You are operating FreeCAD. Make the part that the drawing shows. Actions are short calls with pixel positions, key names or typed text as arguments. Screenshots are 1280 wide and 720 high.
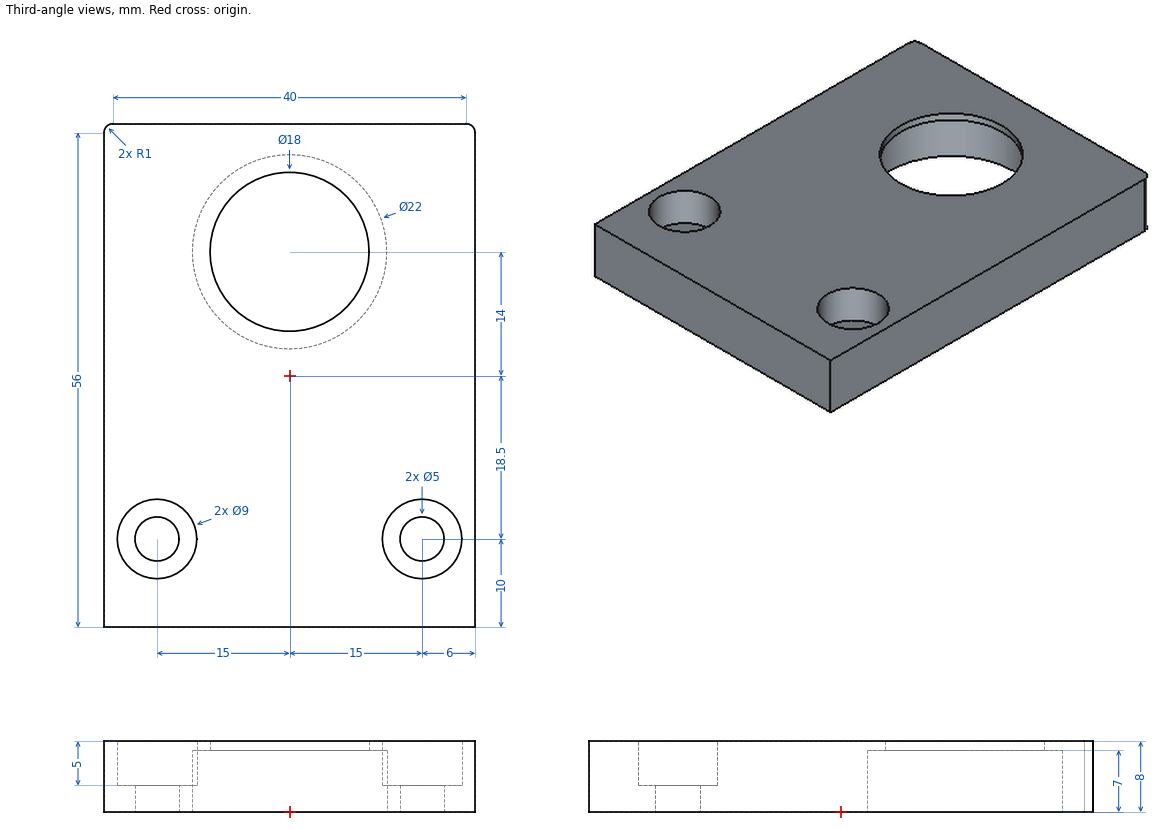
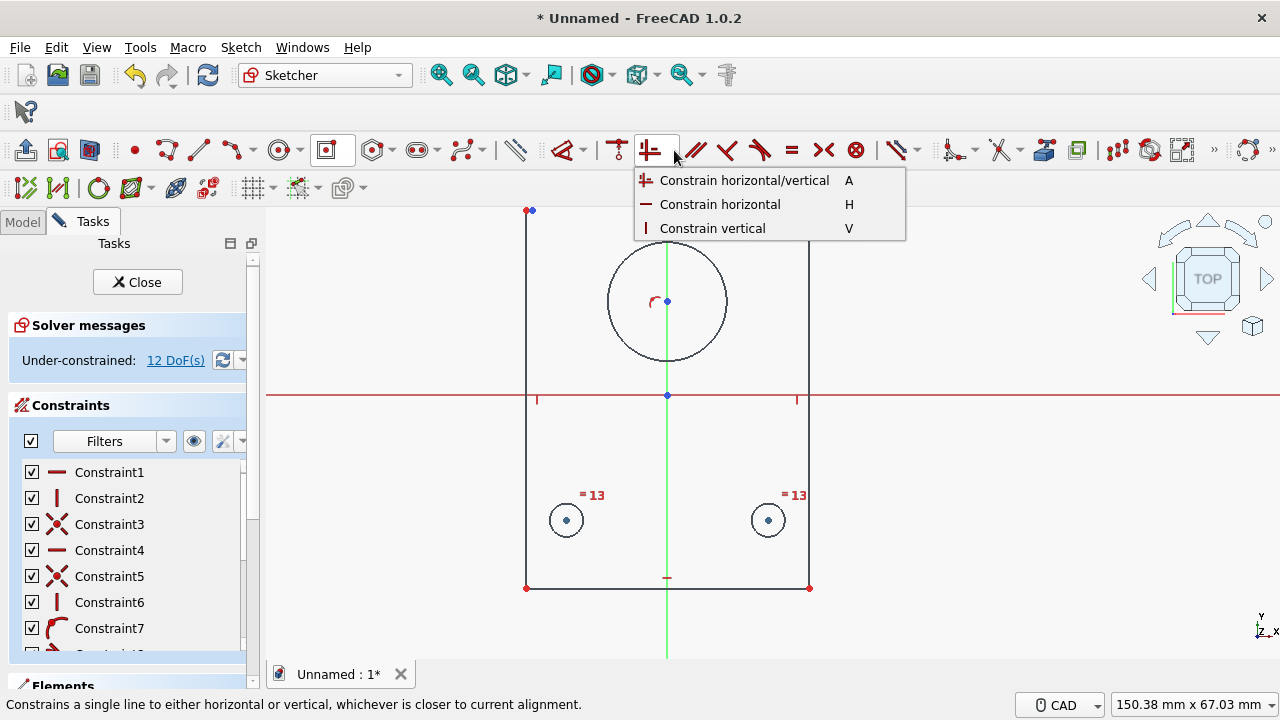
click(770, 204)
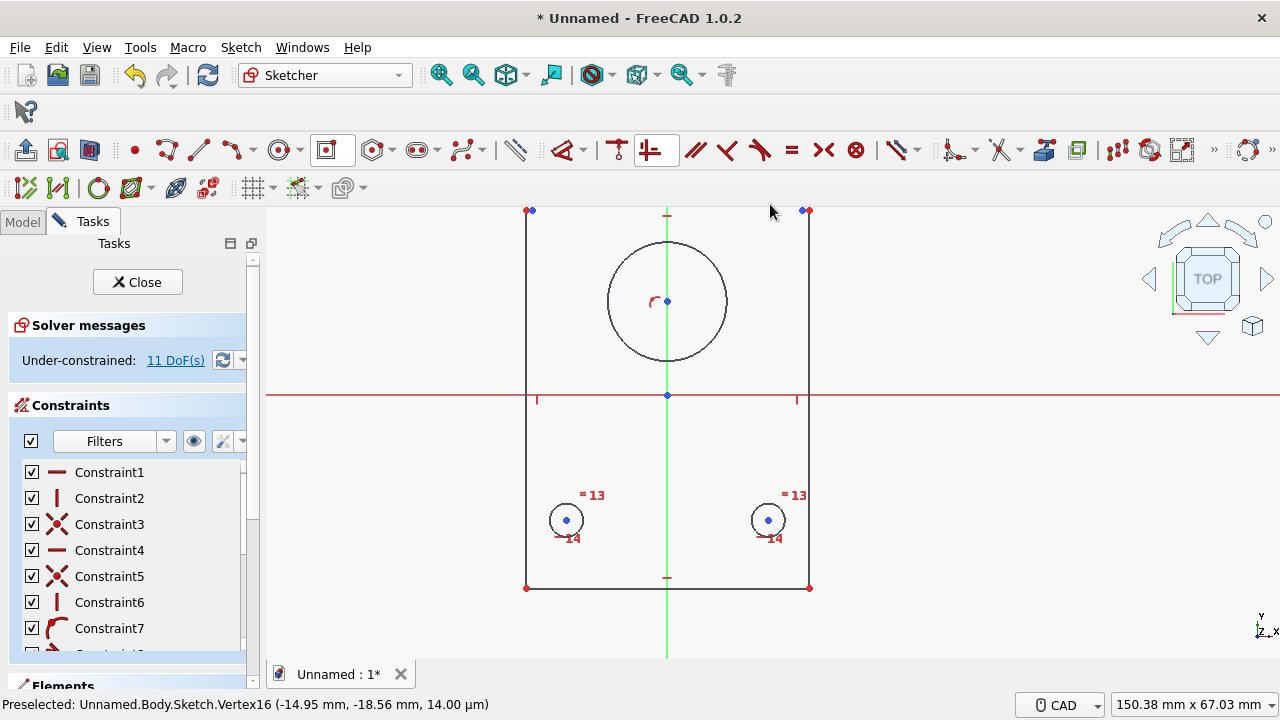
click(562, 150)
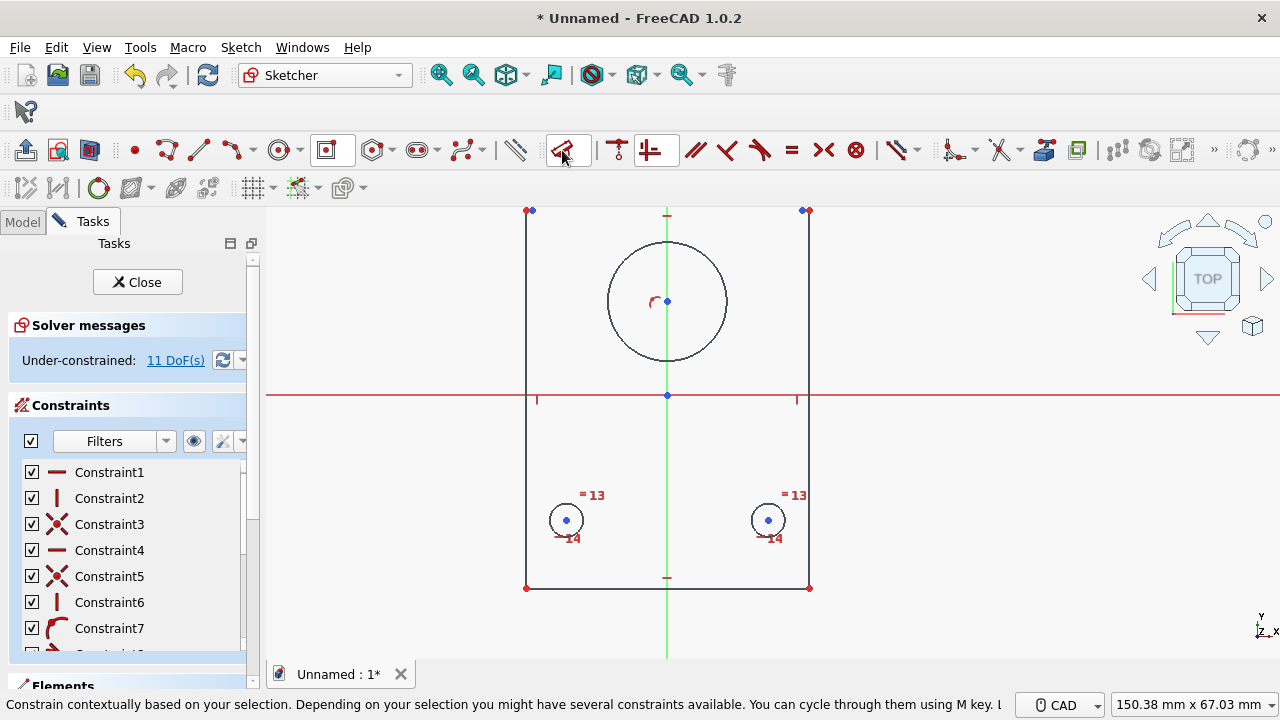
scroll(780, 510, down, 2)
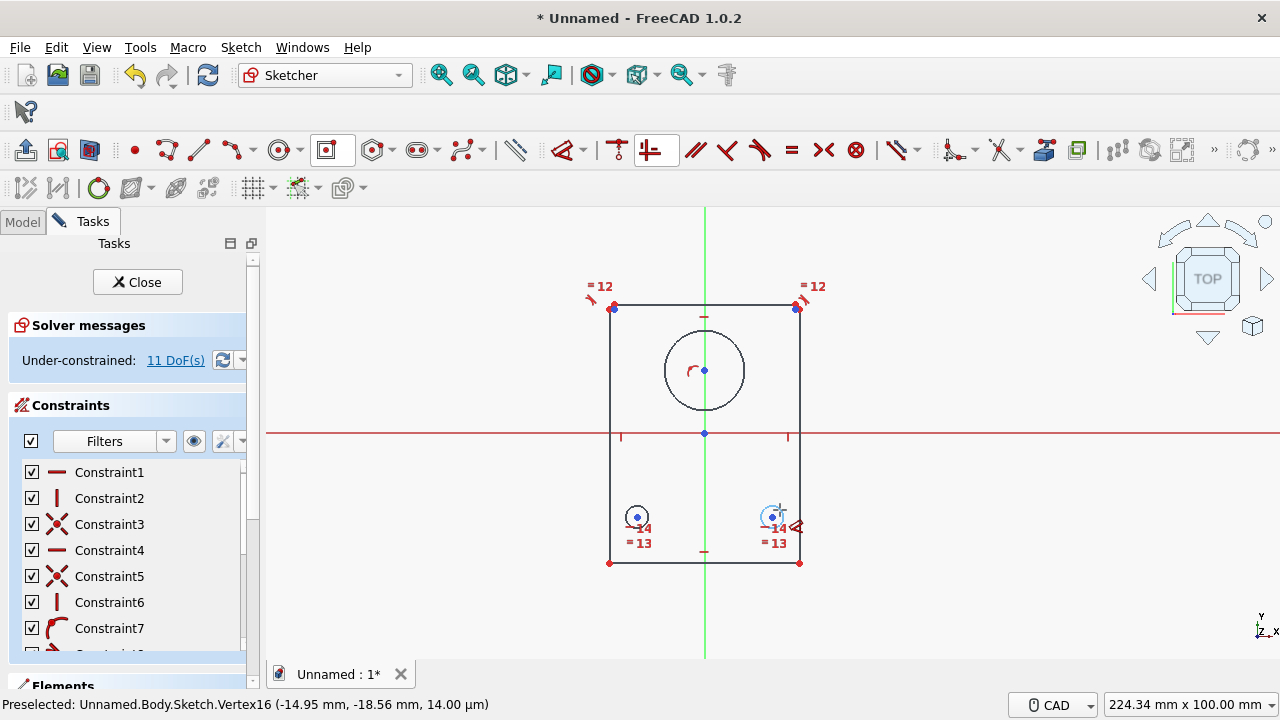
scroll(611, 306, up, 11)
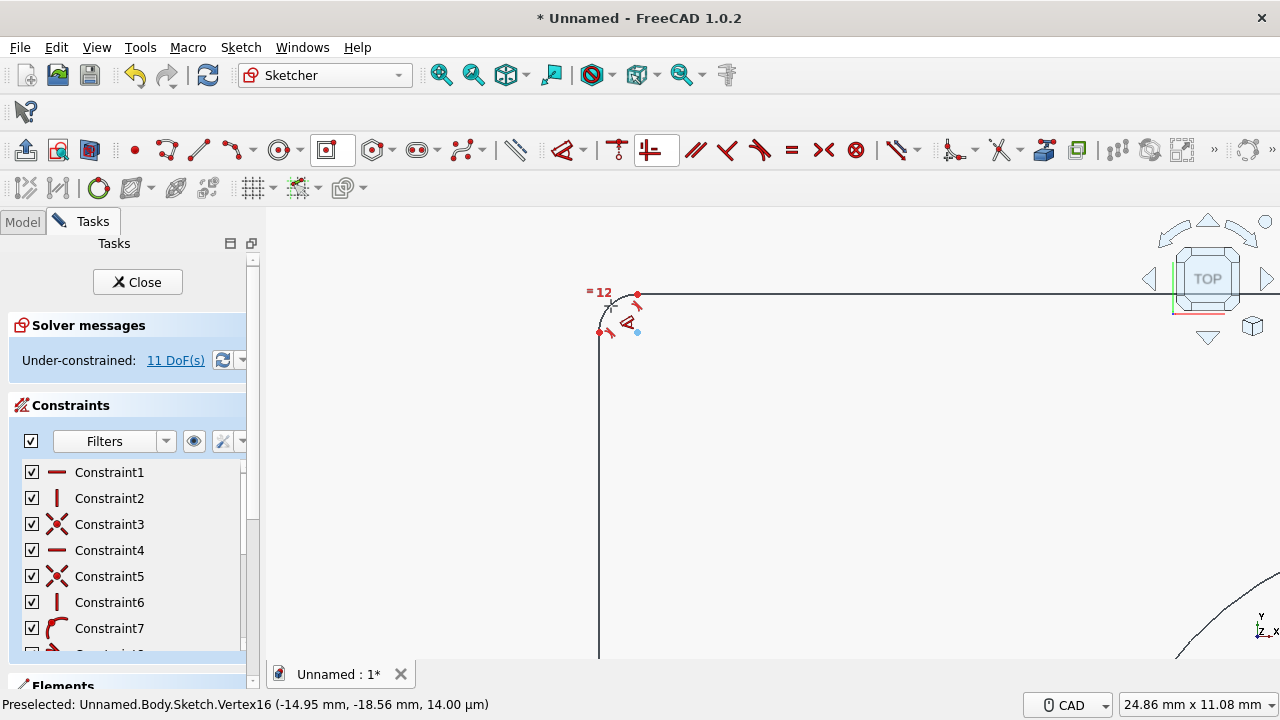
click(610, 306)
click(587, 284)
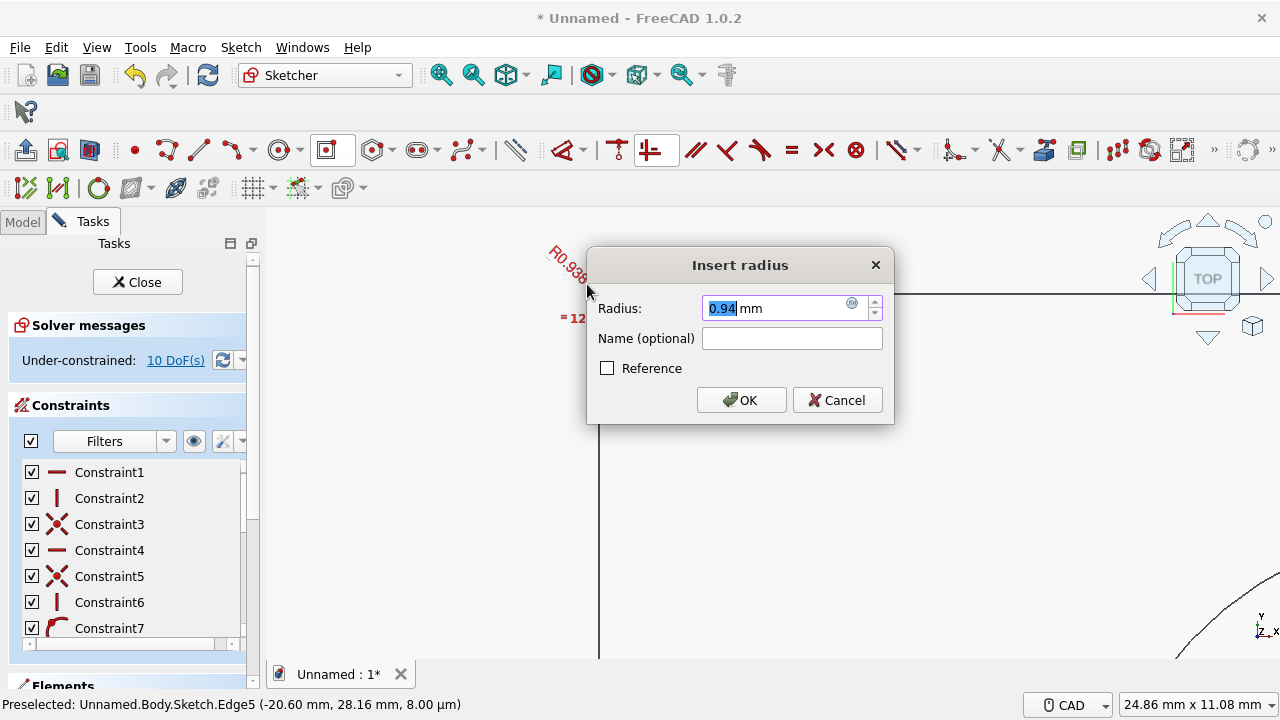
text(1)
key(Return)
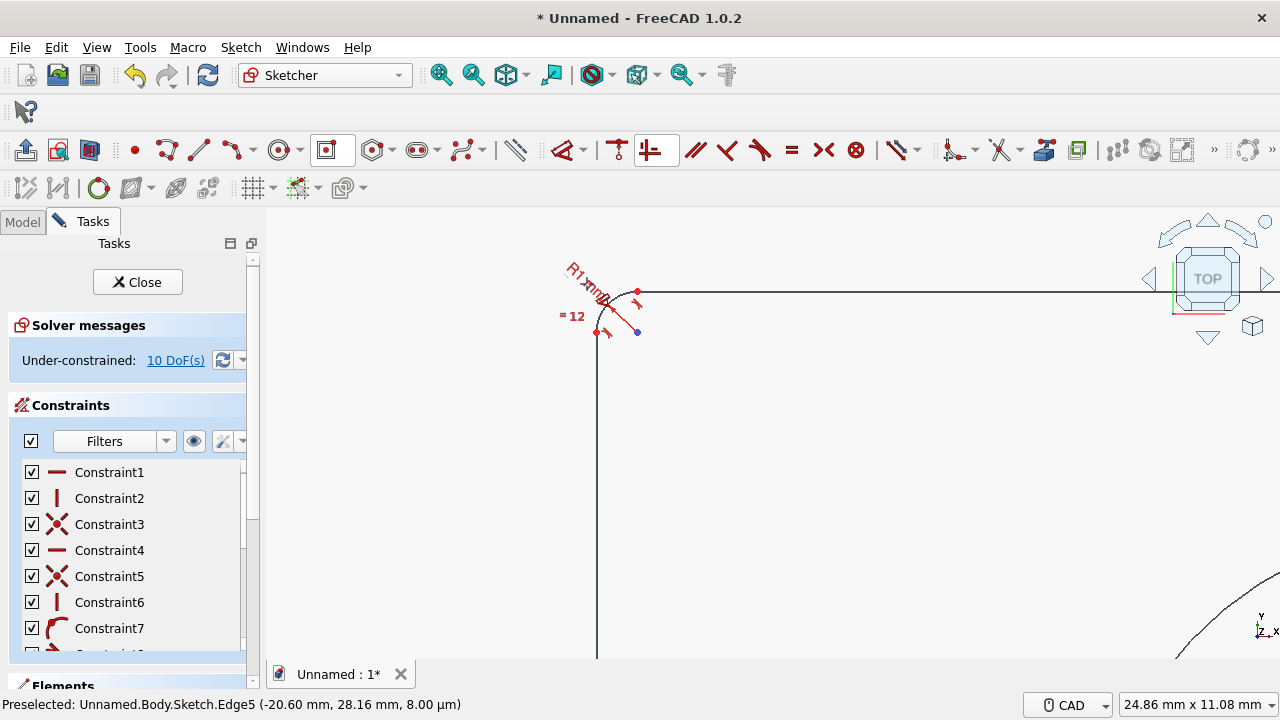
scroll(611, 306, down, 11)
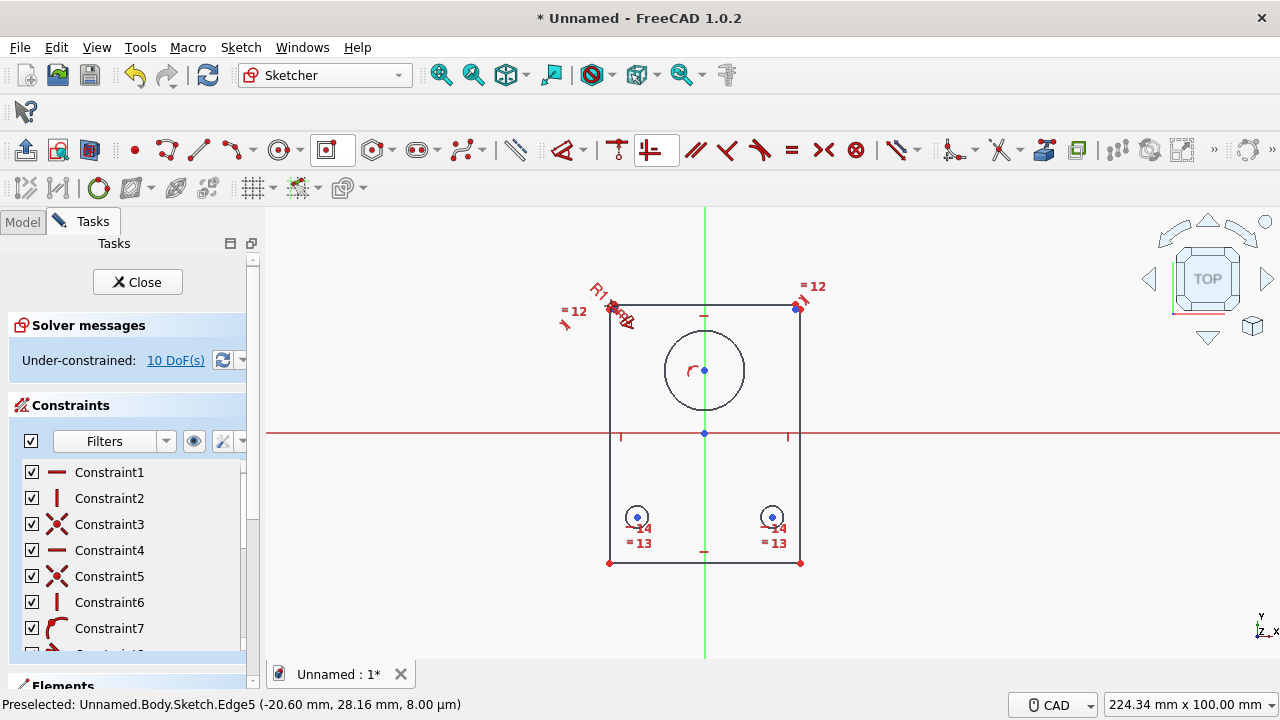
scroll(780, 509, up, 3)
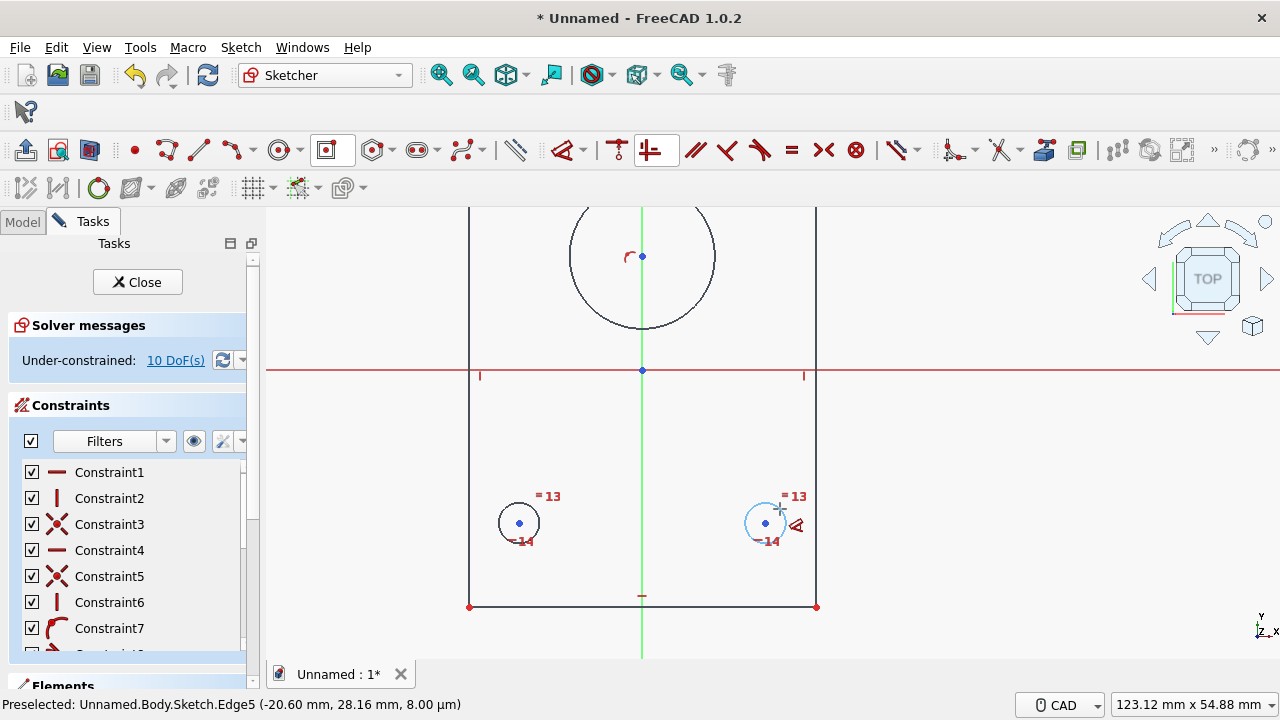
click(780, 509)
click(803, 487)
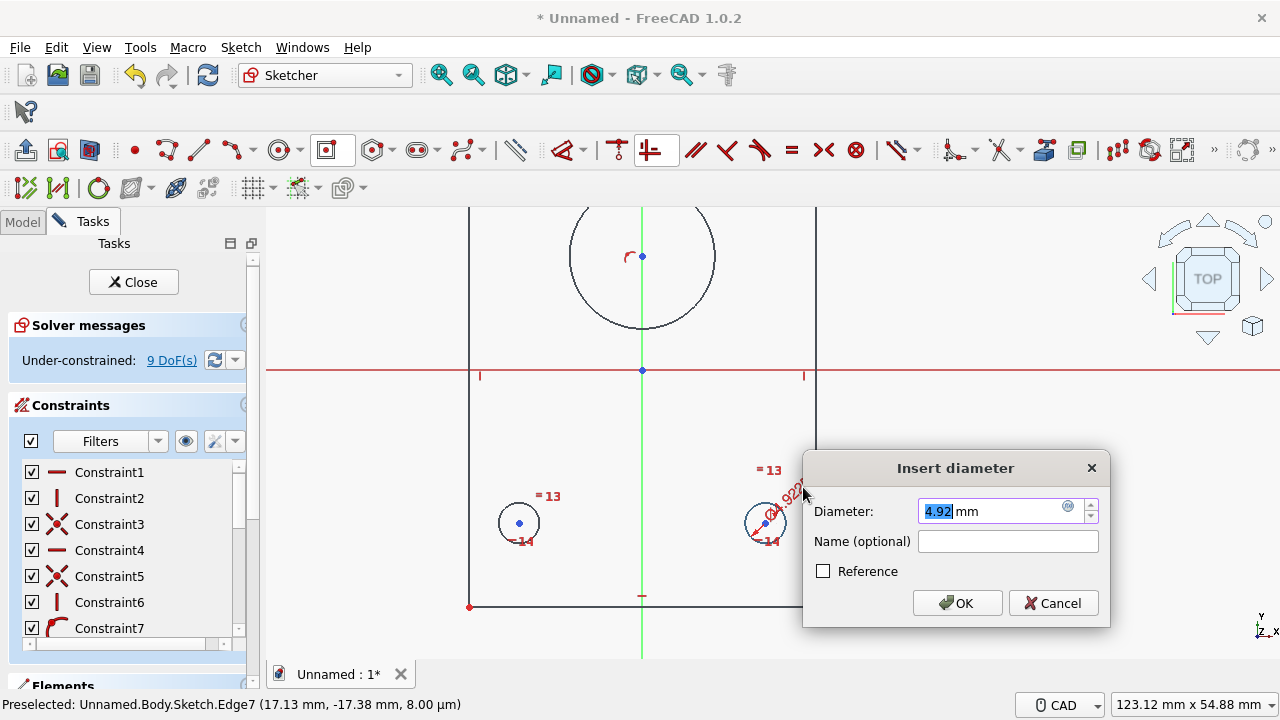
text(5)
key(Return)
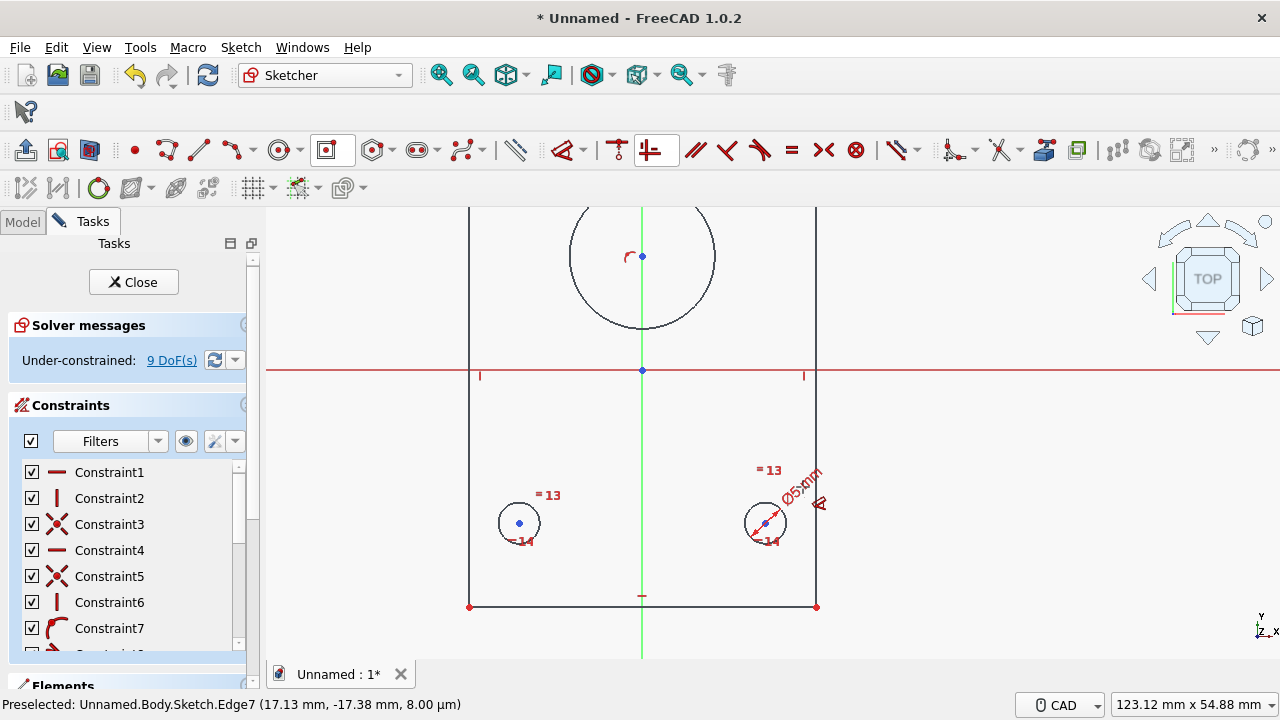
click(591, 308)
click(568, 331)